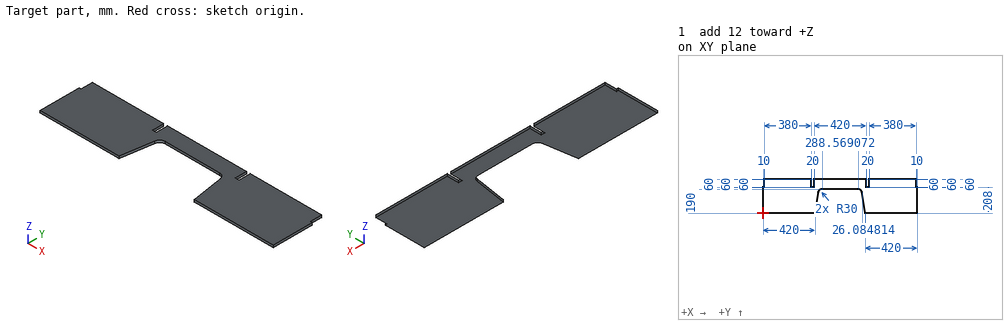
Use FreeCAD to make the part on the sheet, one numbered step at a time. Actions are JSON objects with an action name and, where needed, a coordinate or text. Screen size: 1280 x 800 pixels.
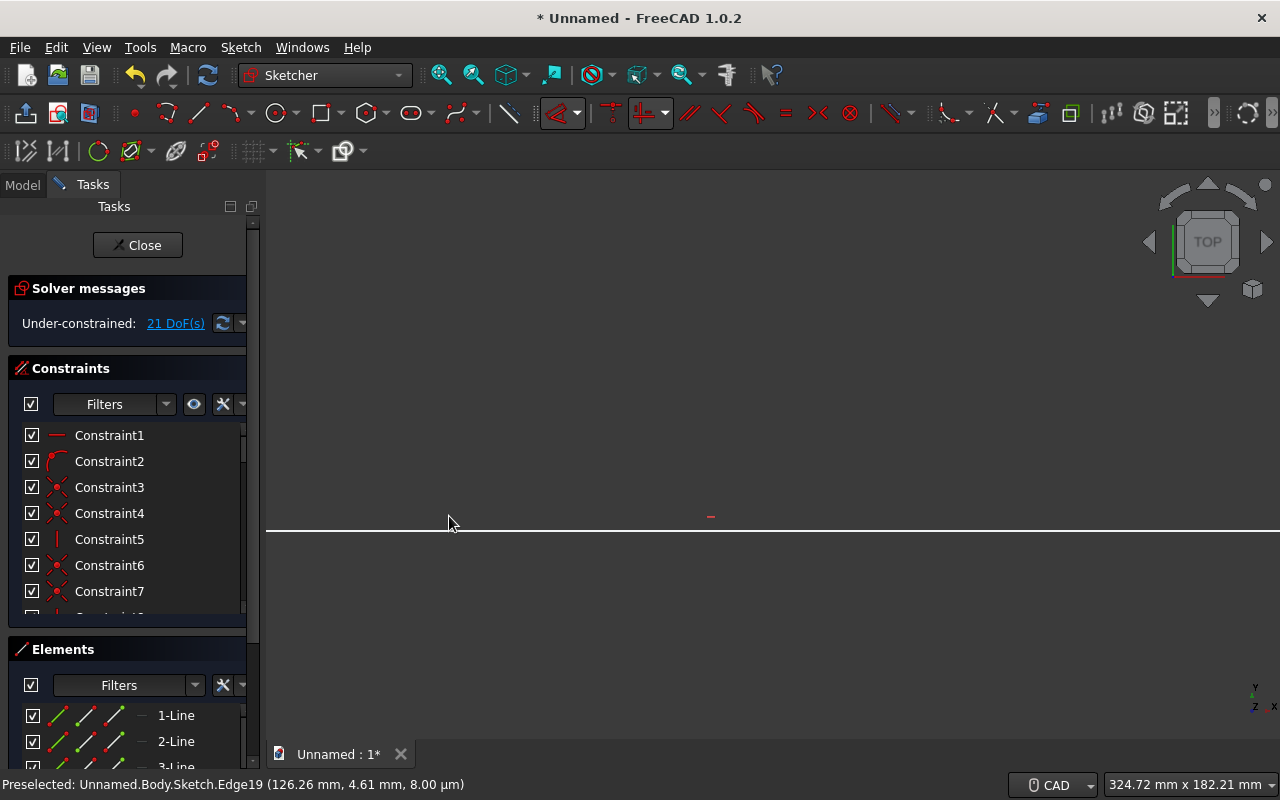
{"action": "scroll", "coordinate": [450, 522], "scroll_direction": "down", "scroll_amount": 9}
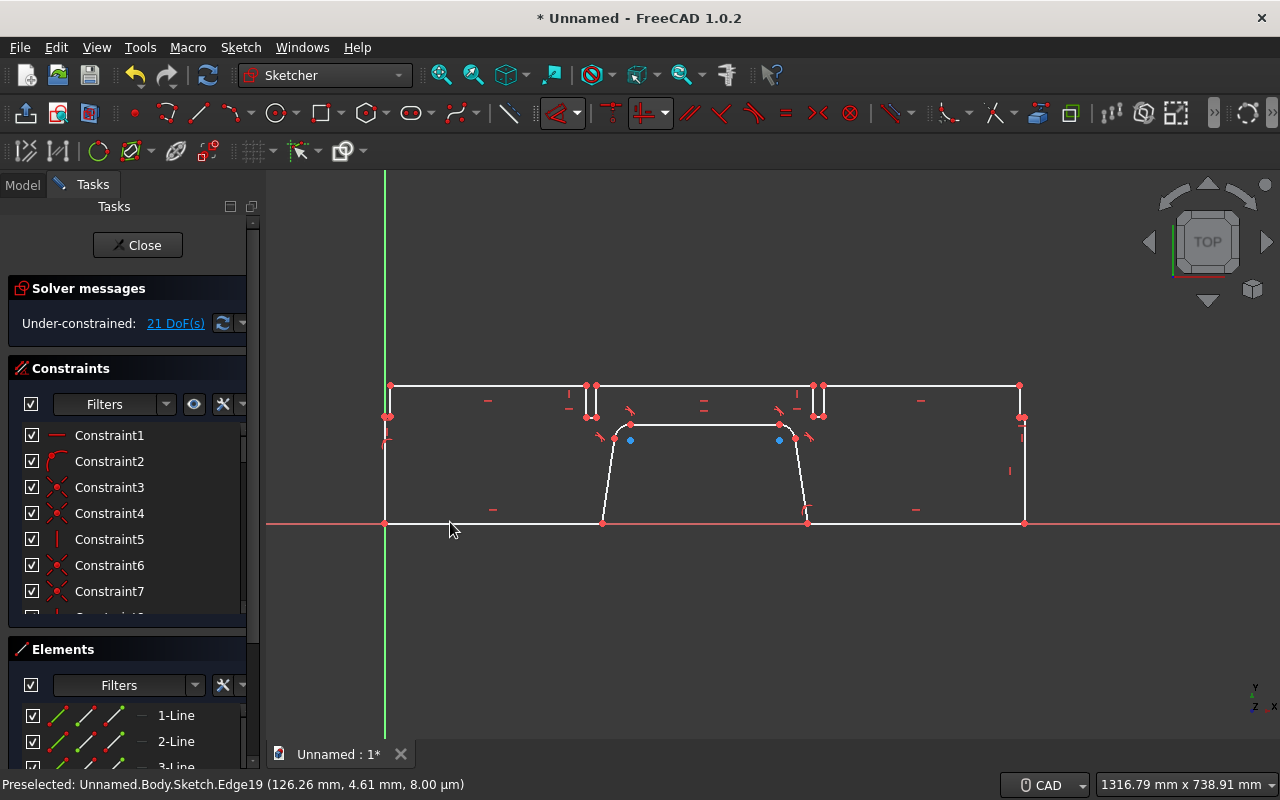
{"action": "scroll", "coordinate": [793, 432], "scroll_direction": "up", "scroll_amount": 4}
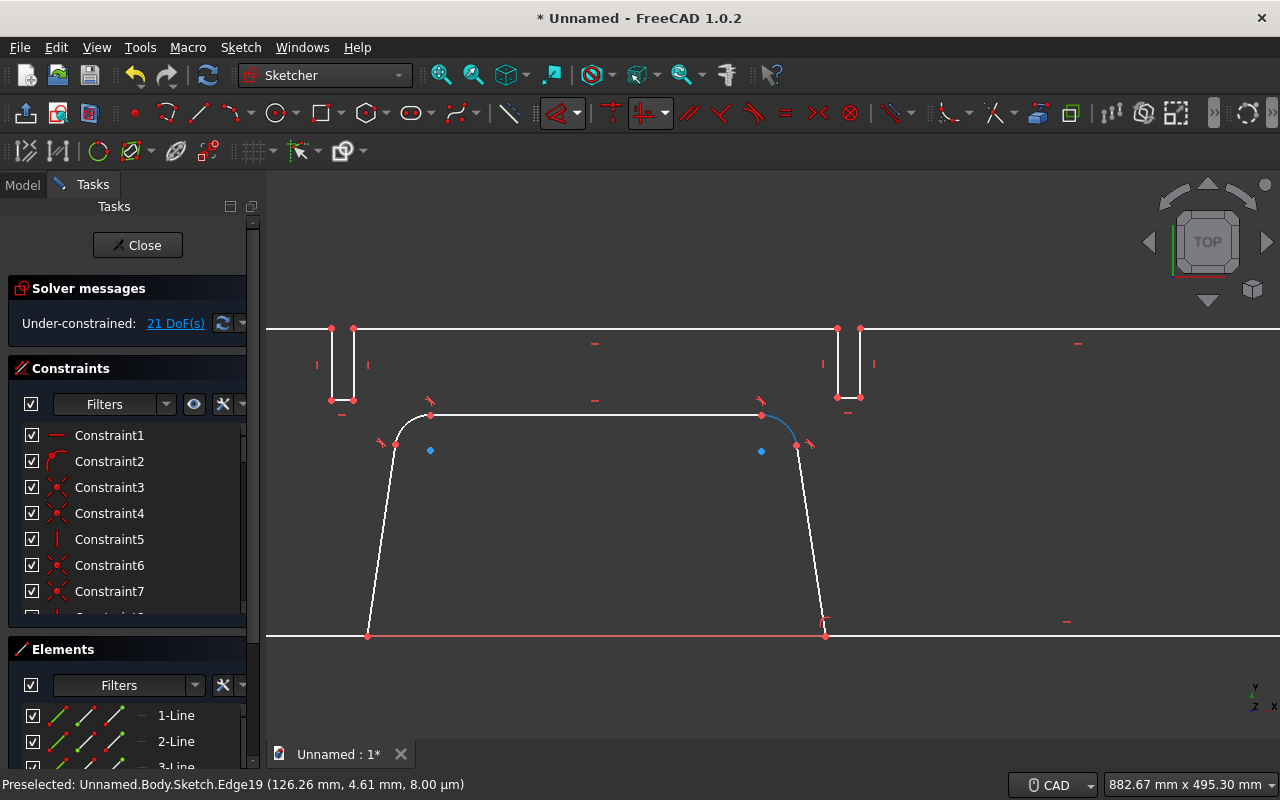
{"action": "left_click", "coordinate": [791, 431]}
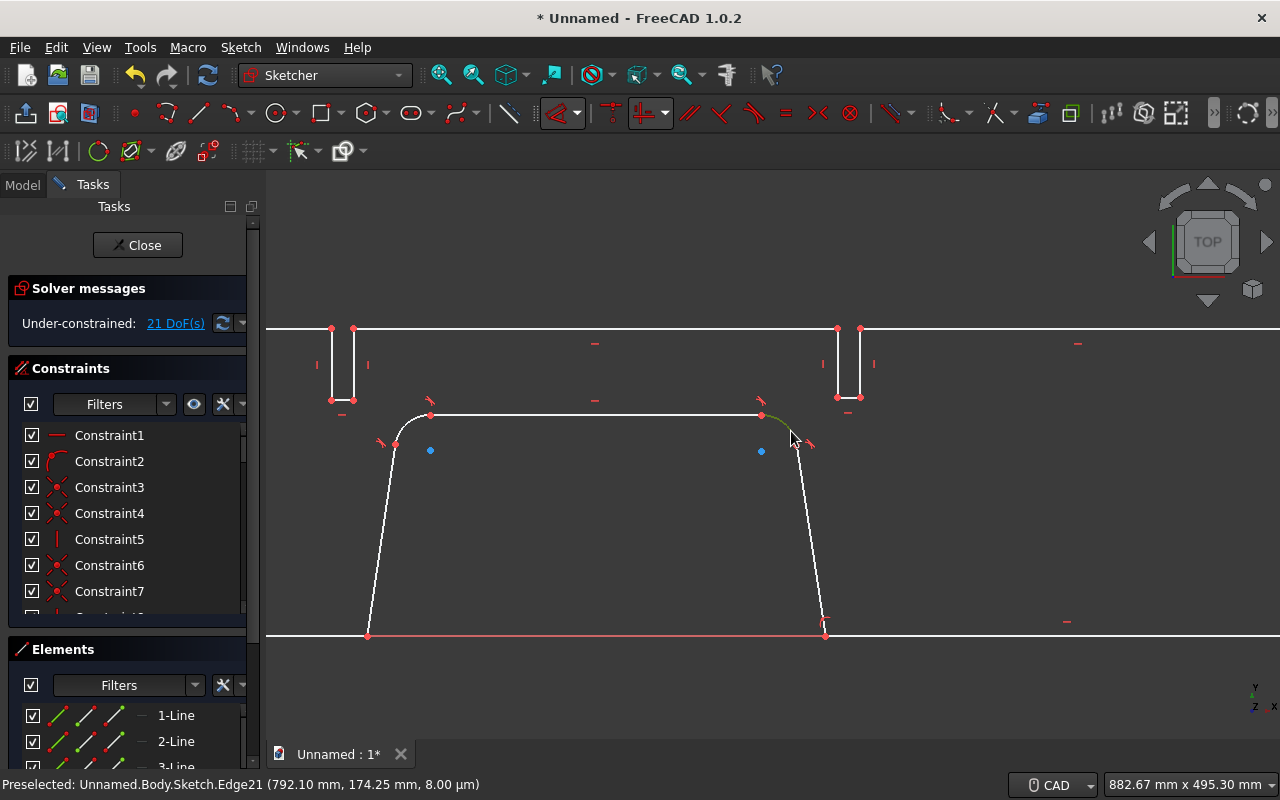
{"action": "left_click", "coordinate": [416, 418]}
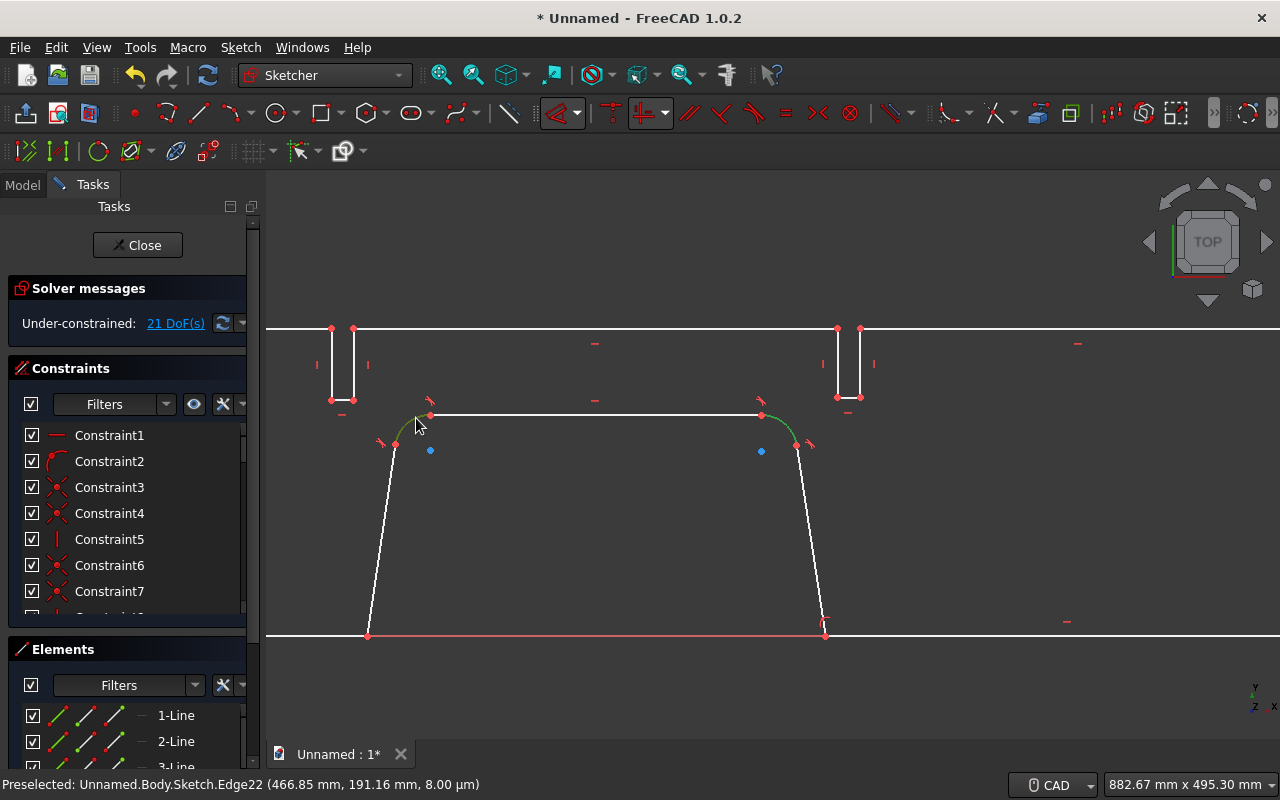
{"action": "key", "text": "e"}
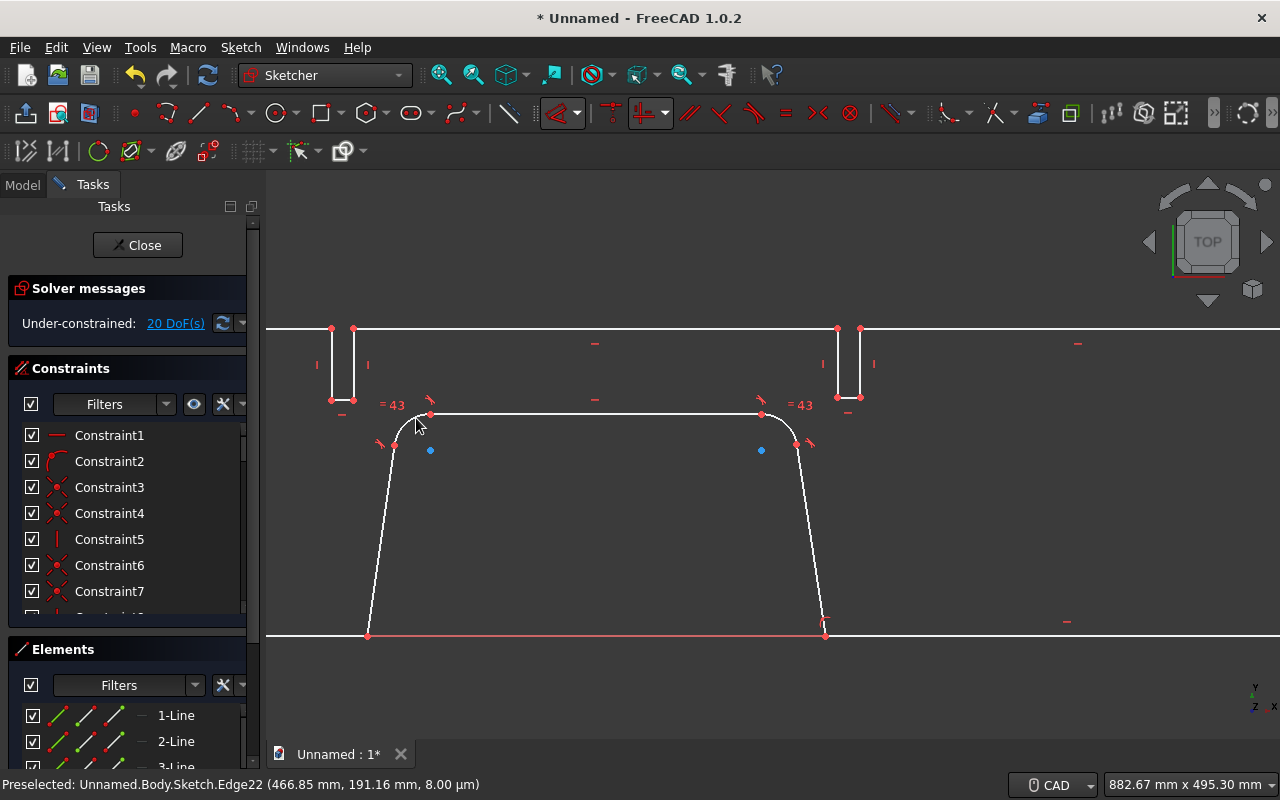
{"action": "key", "text": "d"}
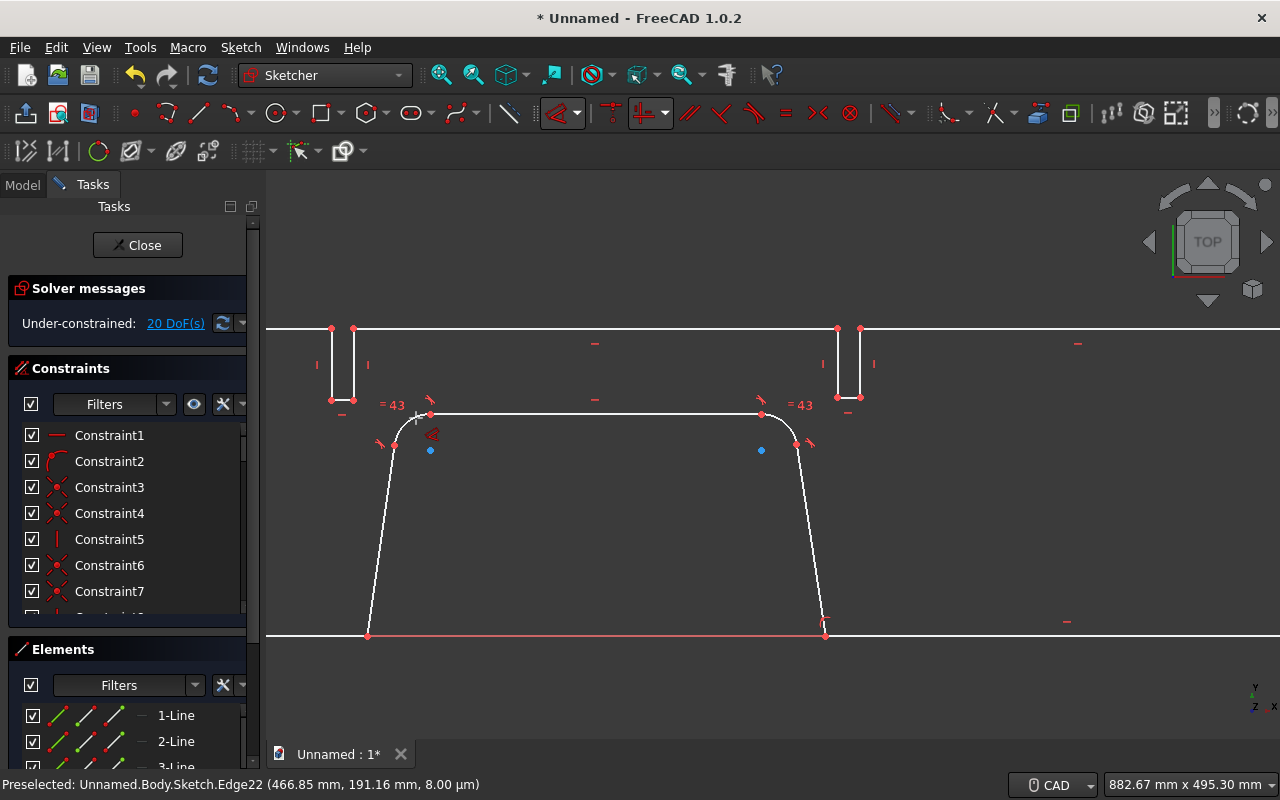
{"action": "left_click", "coordinate": [791, 431]}
{"action": "left_click", "coordinate": [818, 414]}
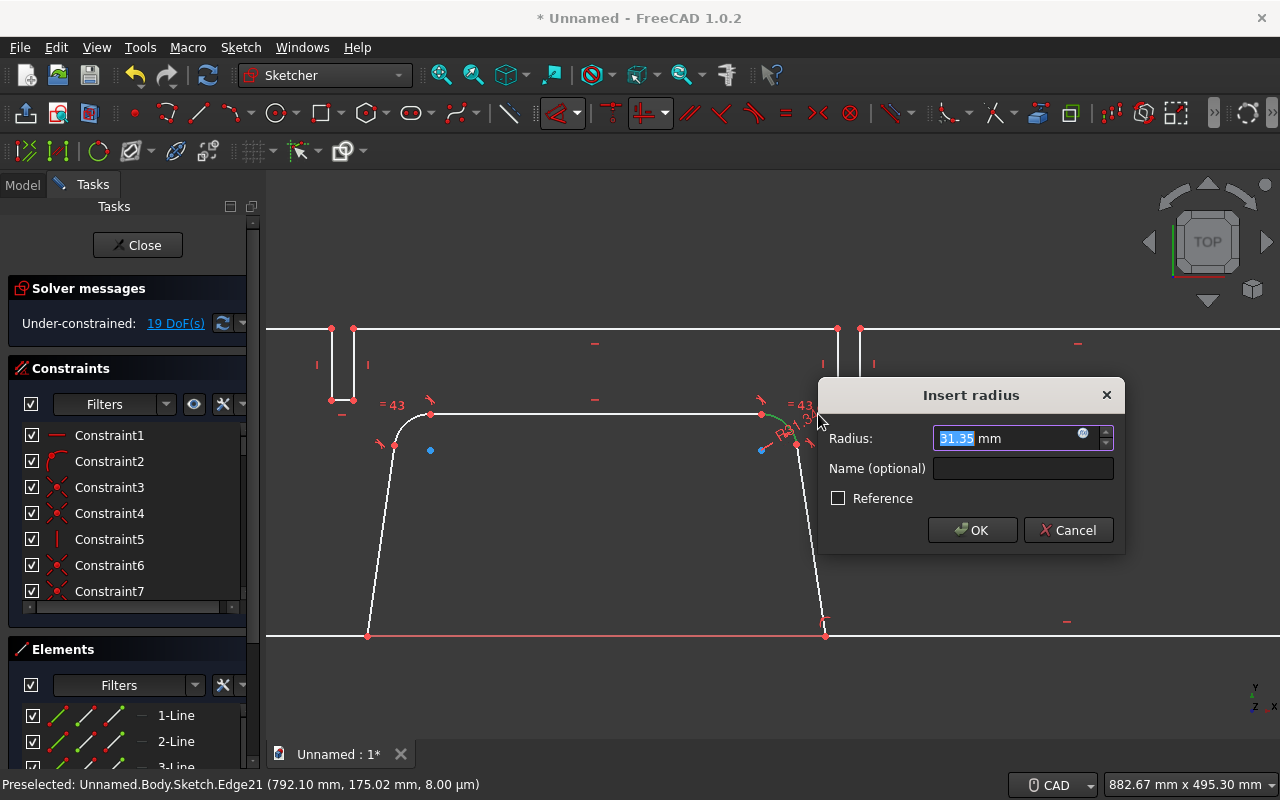
{"action": "type", "text": "30"}
{"action": "key", "text": "Return"}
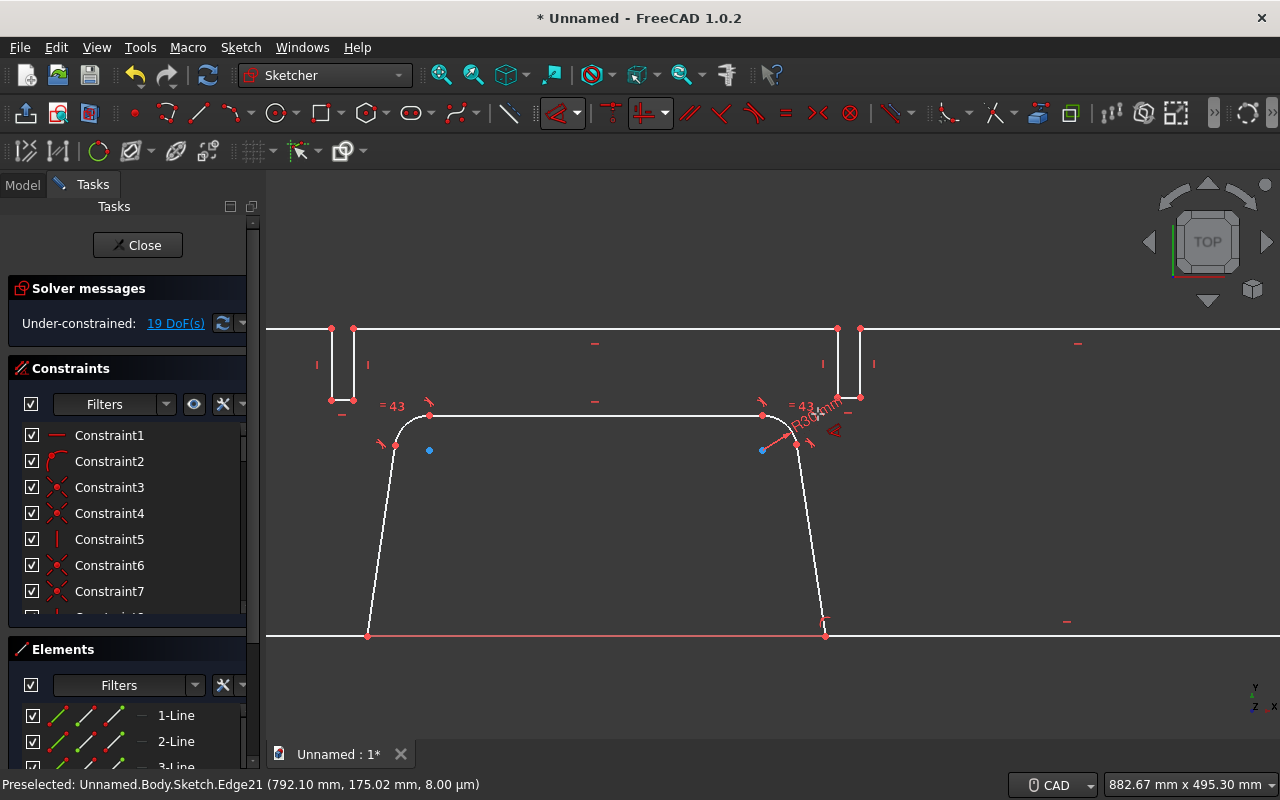
{"action": "scroll", "coordinate": [793, 432], "scroll_direction": "down", "scroll_amount": 4}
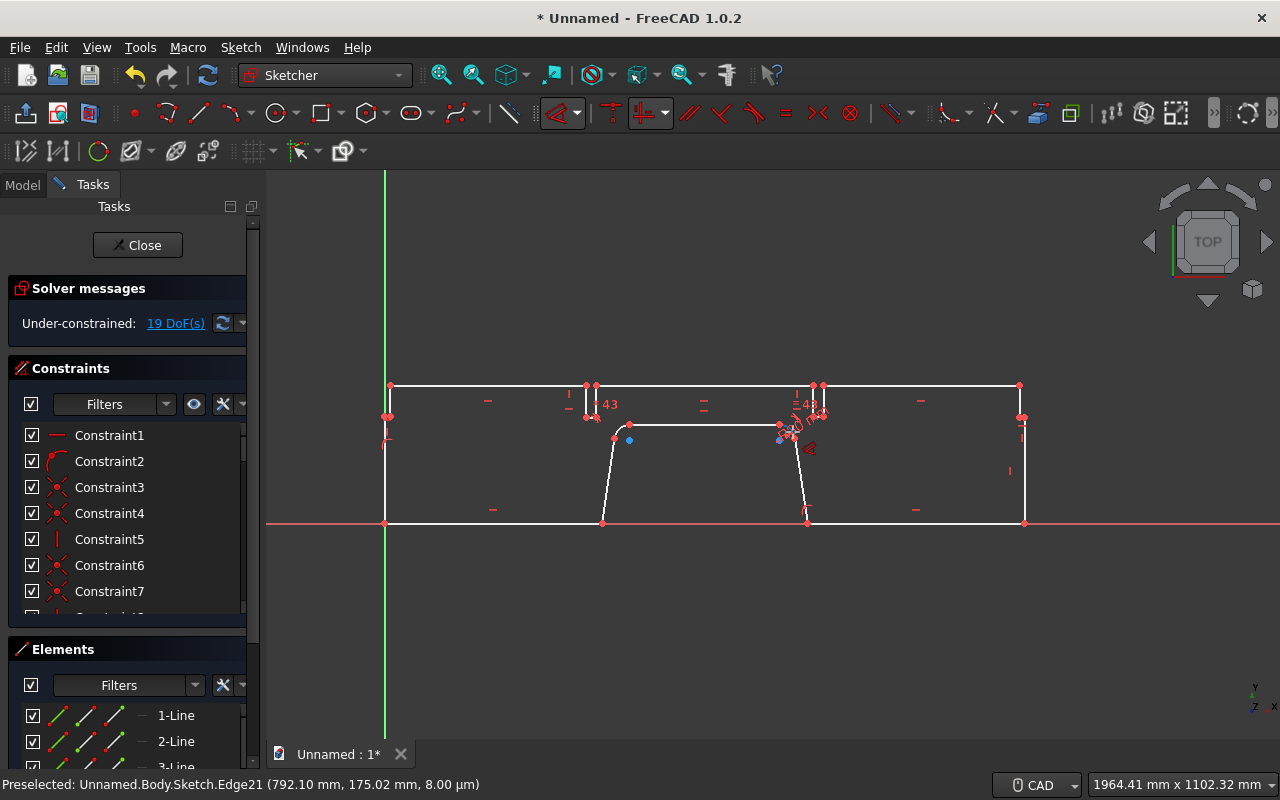
{"action": "scroll", "coordinate": [1022, 417], "scroll_direction": "up", "scroll_amount": 11}